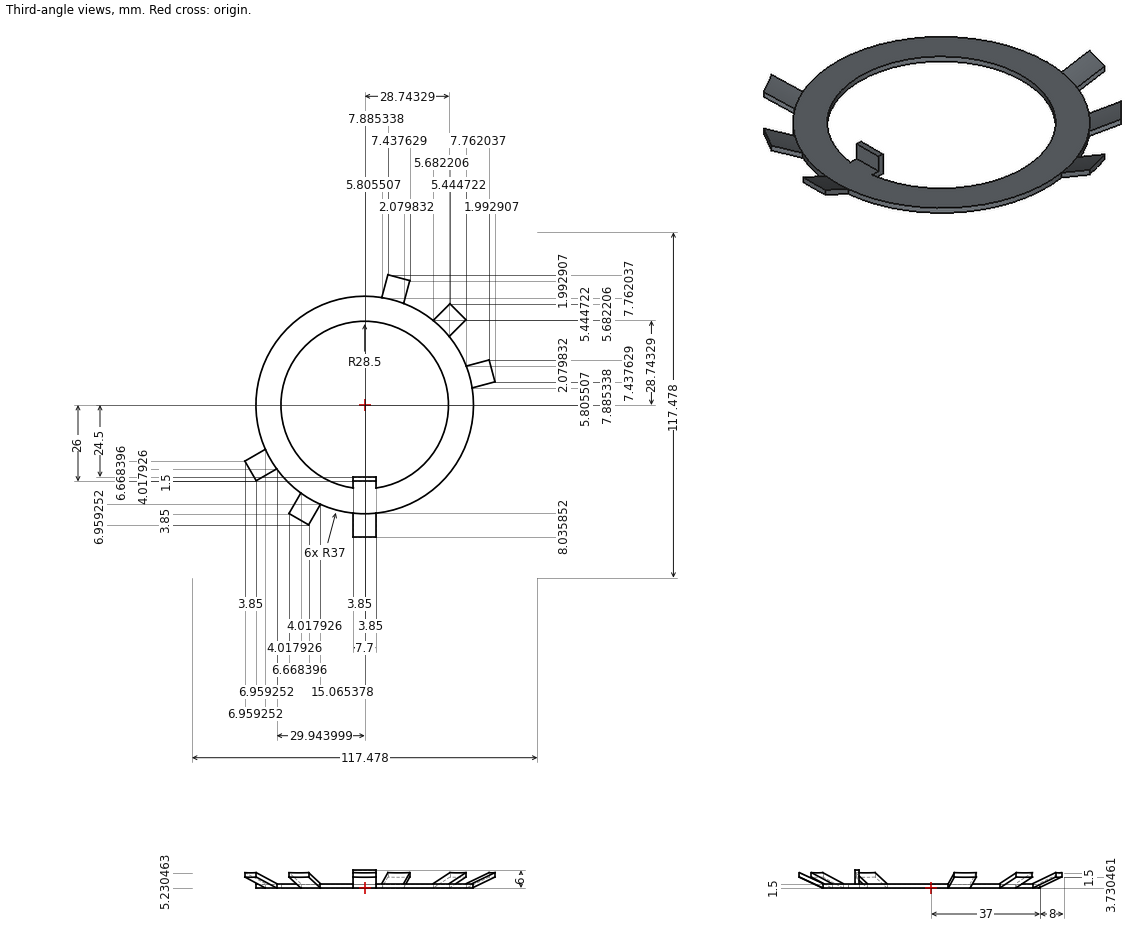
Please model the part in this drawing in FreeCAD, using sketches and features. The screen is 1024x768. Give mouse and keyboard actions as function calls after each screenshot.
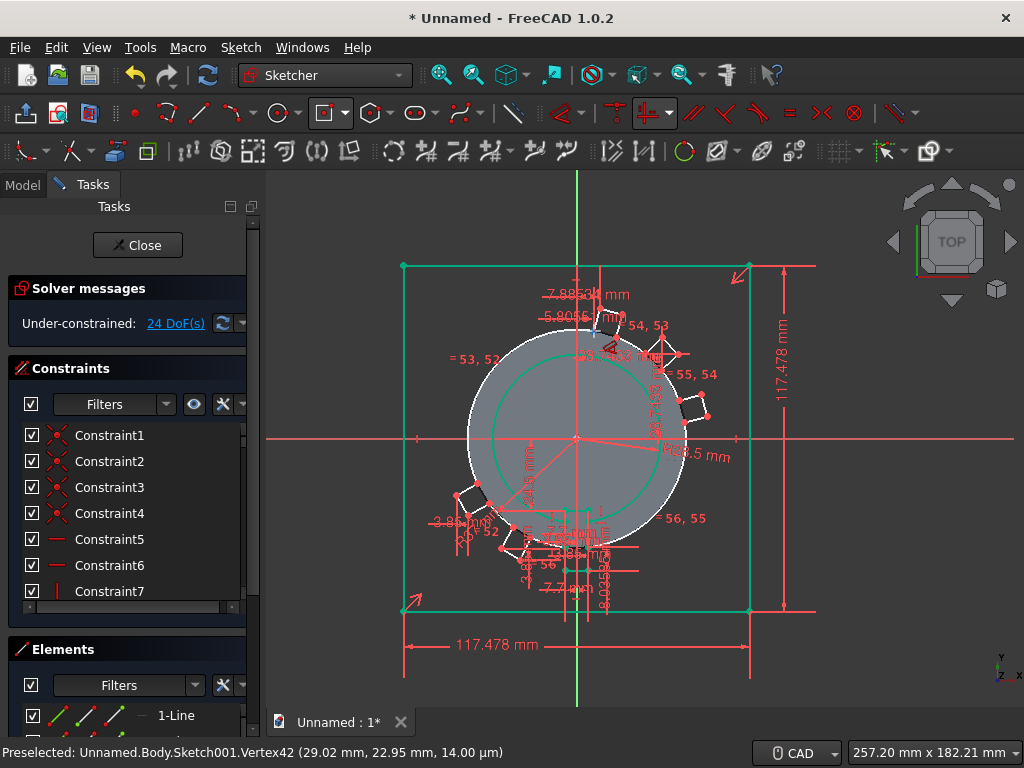
scroll(707, 417, up, 3)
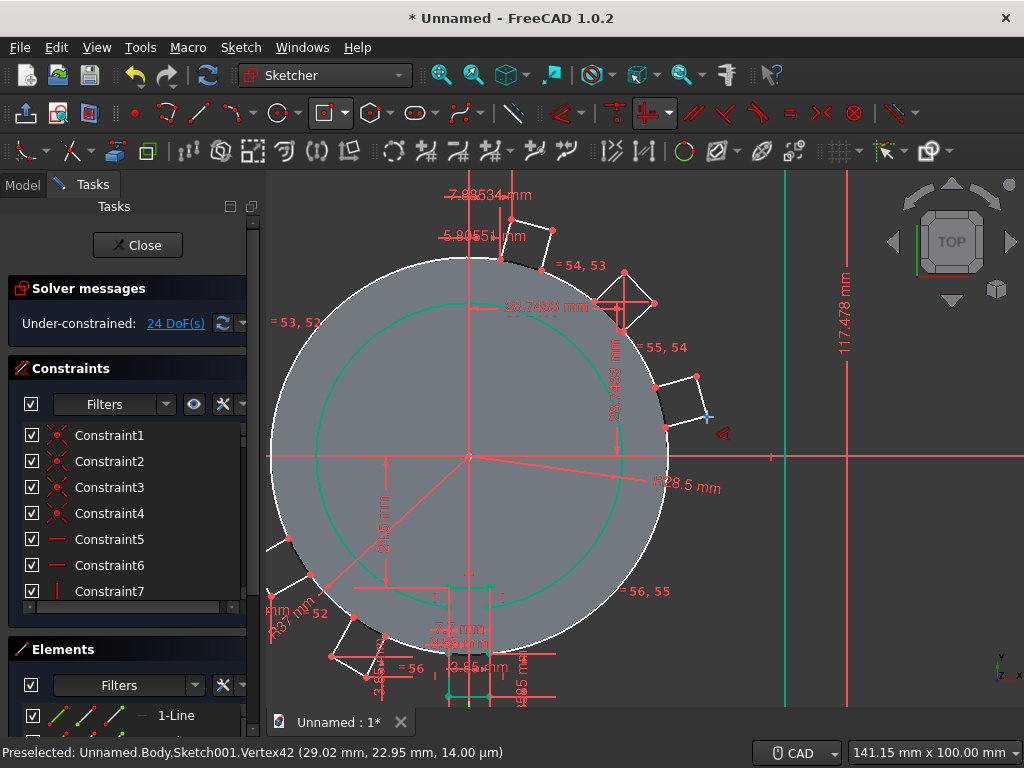
click(707, 416)
click(741, 436)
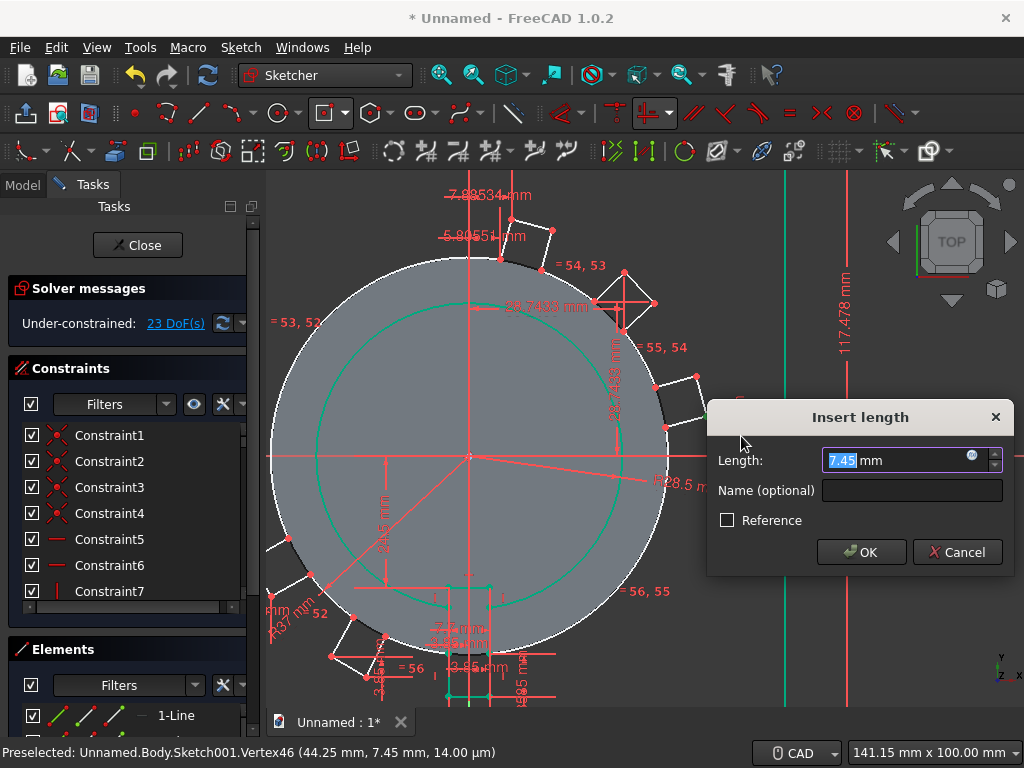
text(7.885338)
key(Return)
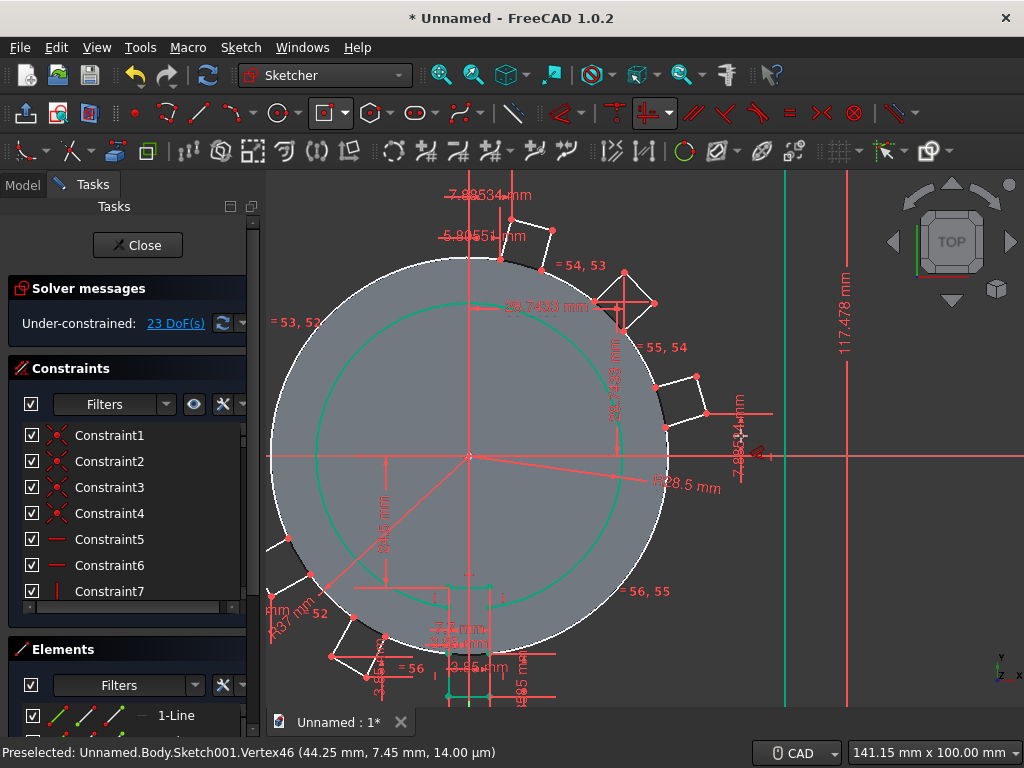
scroll(666, 427, up, 2)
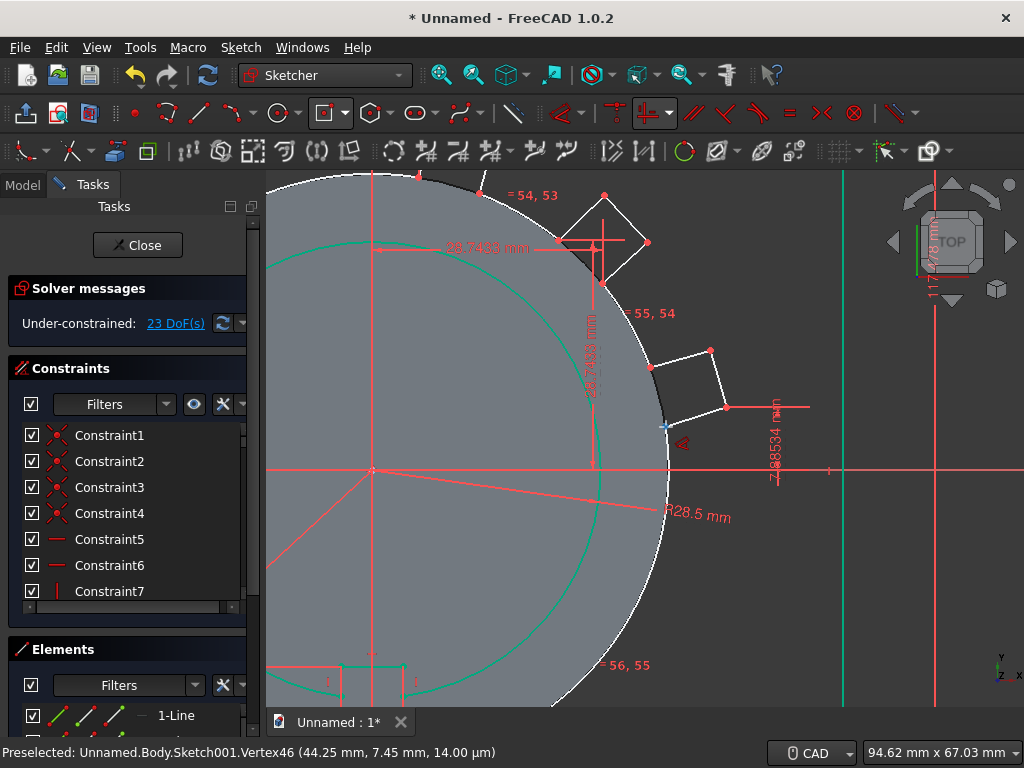
click(666, 427)
click(700, 449)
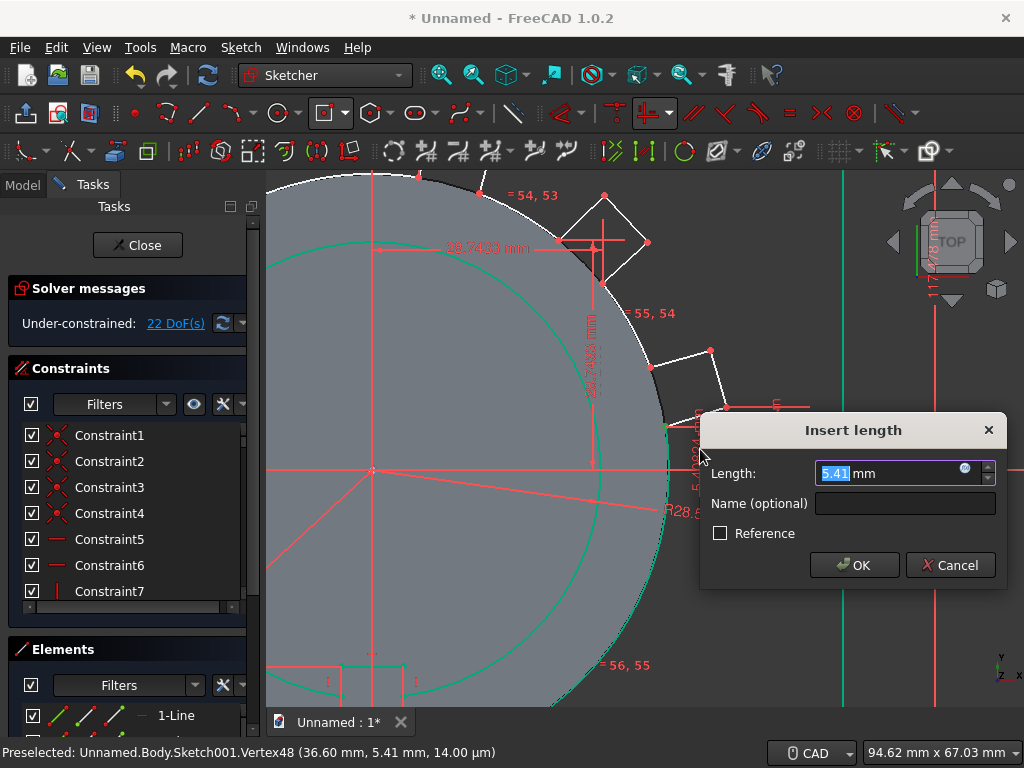
text(5.805507)
key(Return)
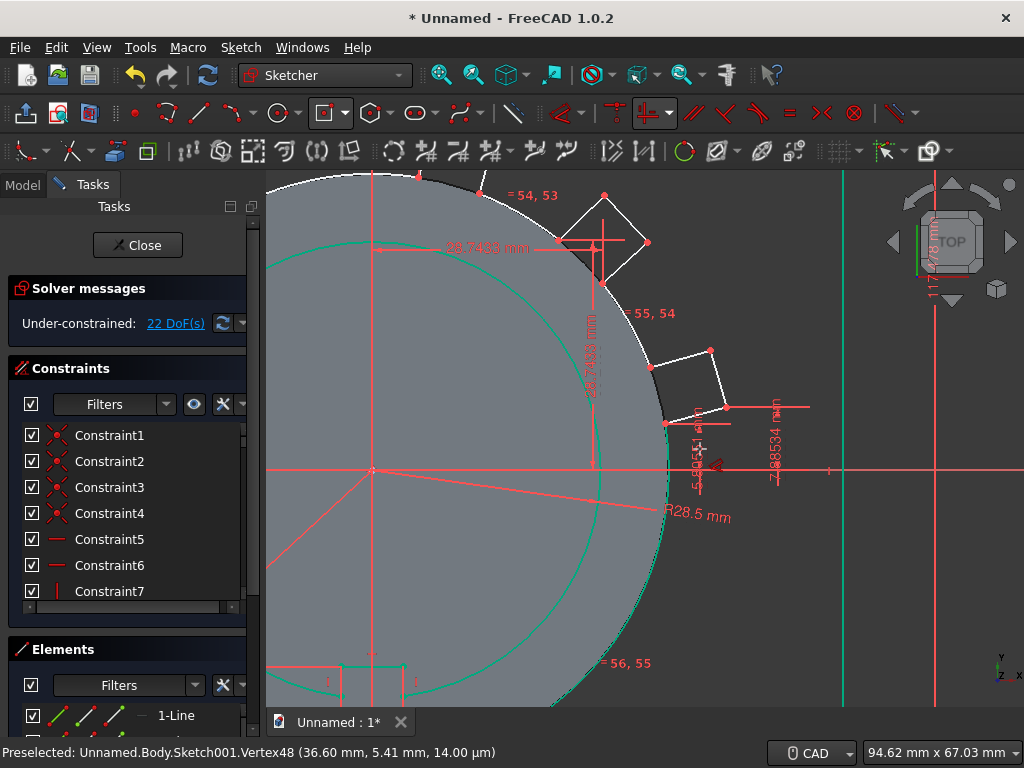
scroll(695, 420, down, 5)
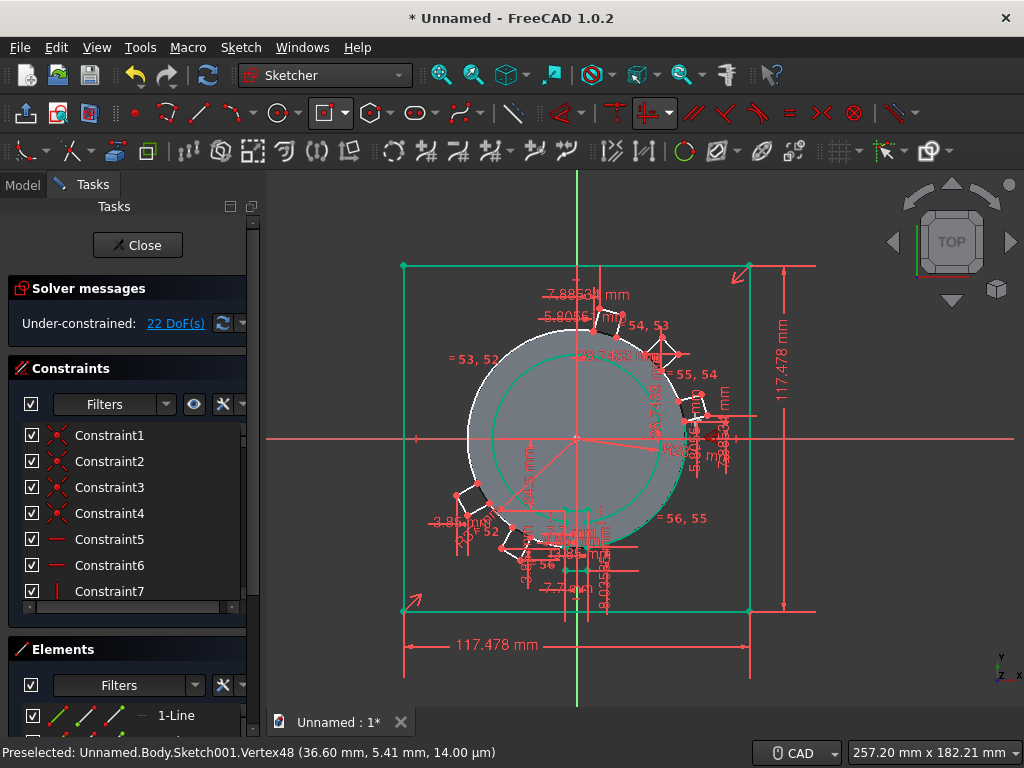
scroll(528, 544, up, 7)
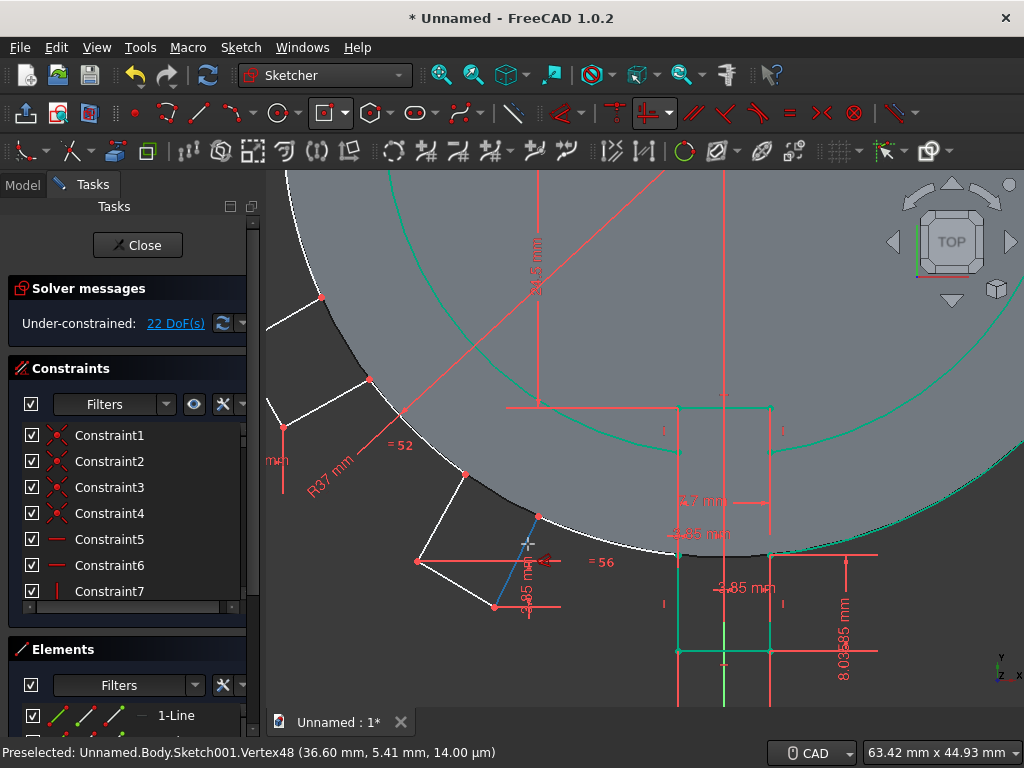
click(525, 544)
click(517, 641)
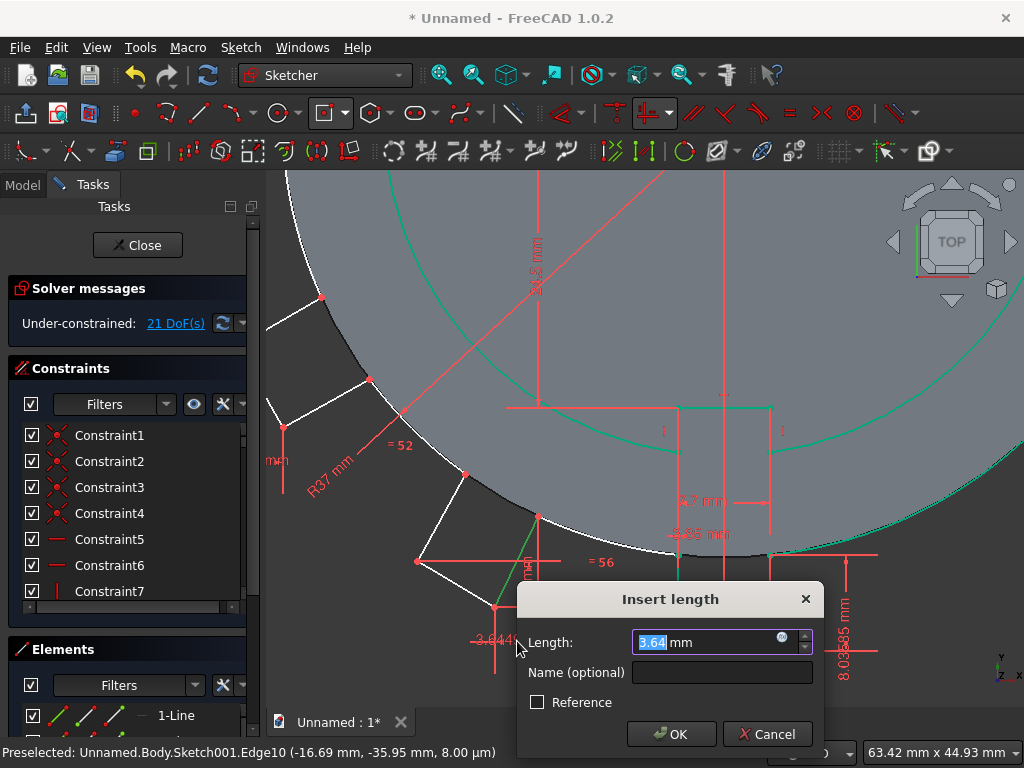
text(4.017926)
key(Return)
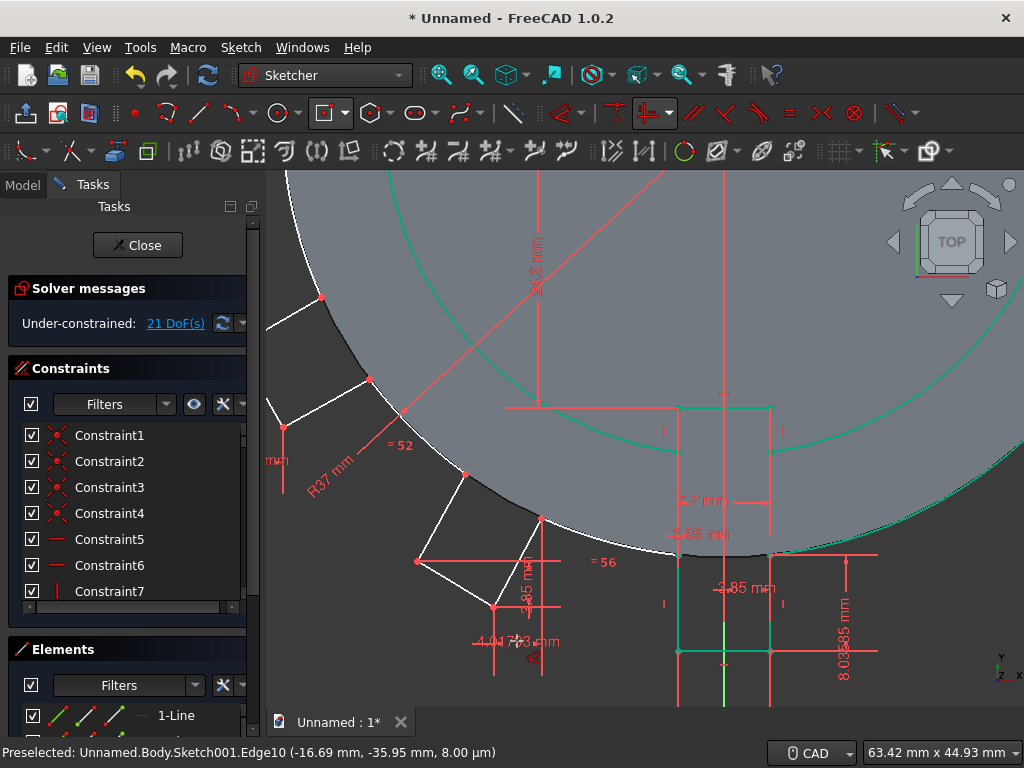
click(528, 545)
click(460, 563)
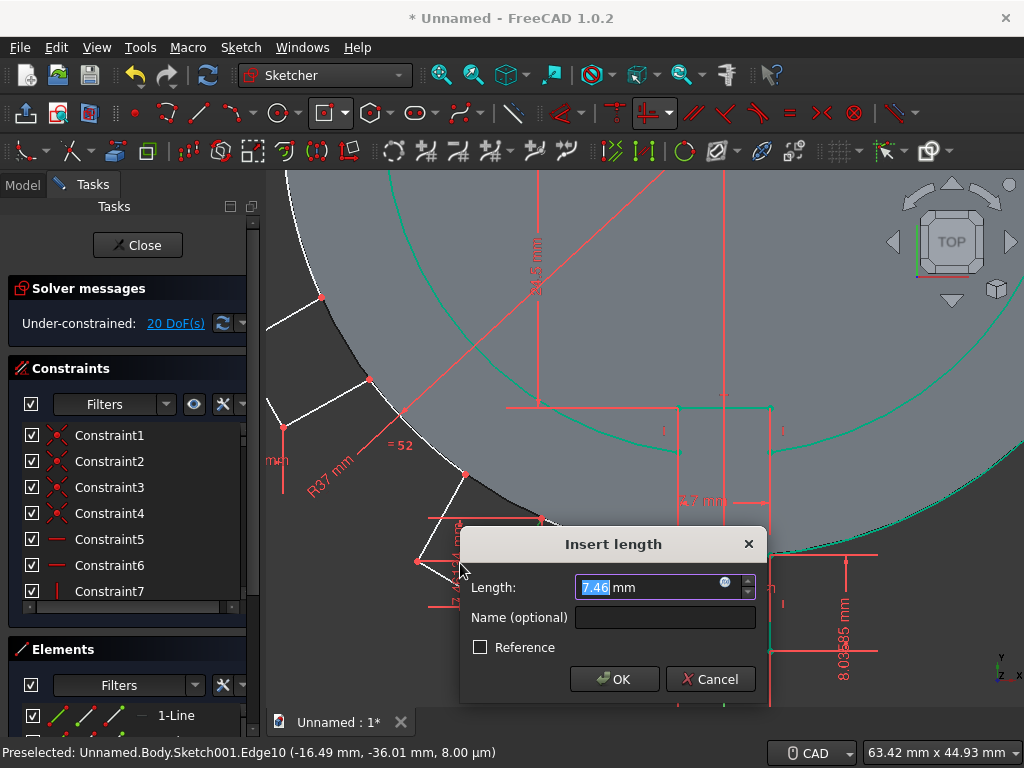
text(6.959252)
key(Return)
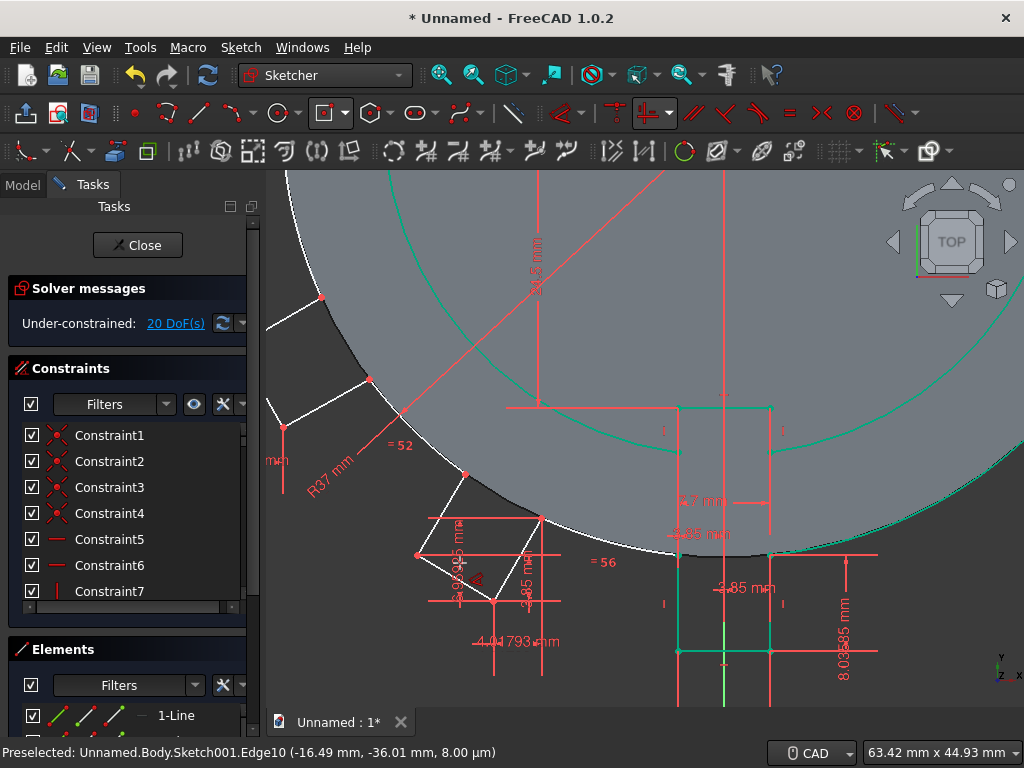
click(471, 587)
click(438, 635)